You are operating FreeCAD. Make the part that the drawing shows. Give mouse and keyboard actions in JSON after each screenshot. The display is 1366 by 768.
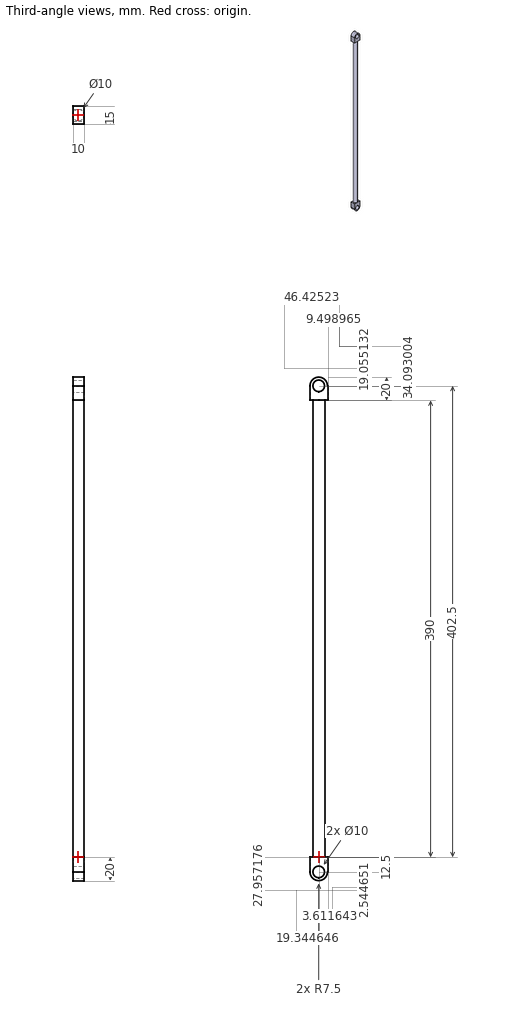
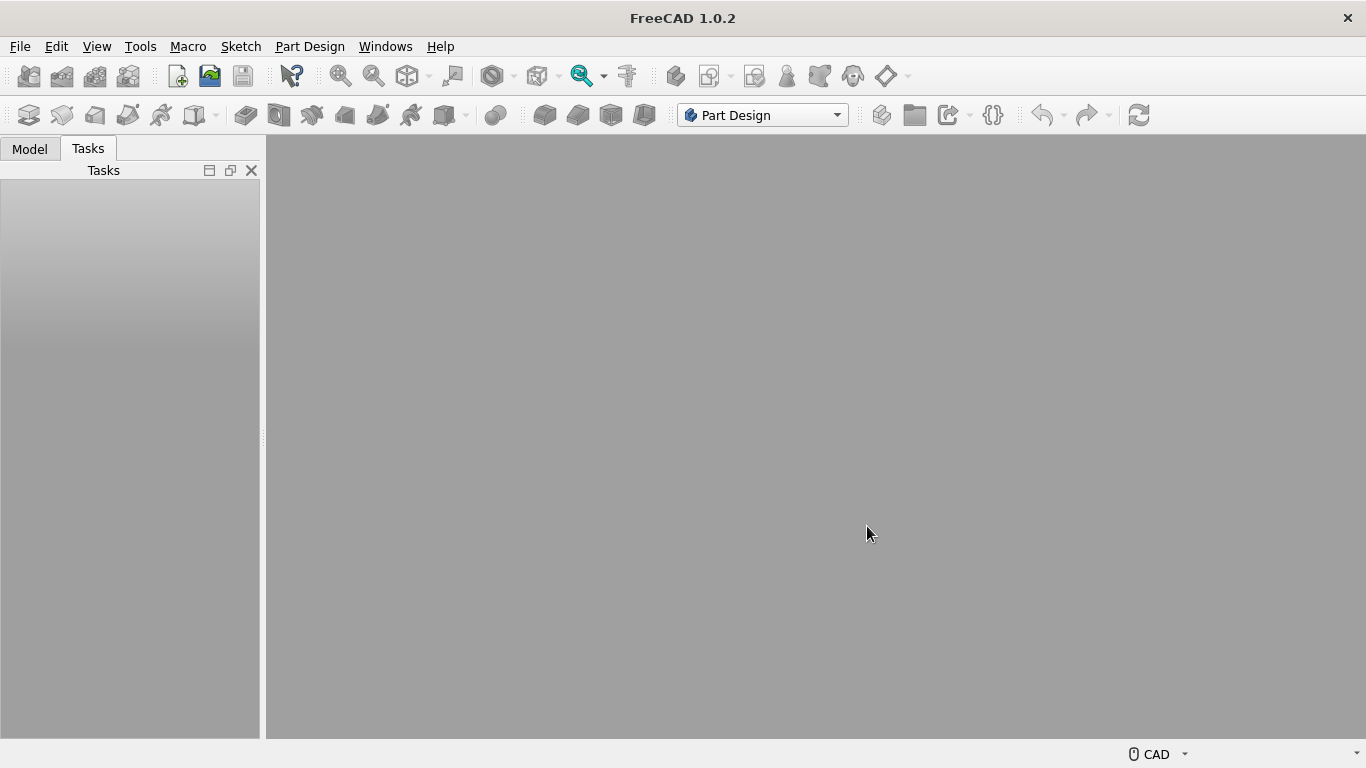
{"action": "left_click", "coordinate": [177, 76]}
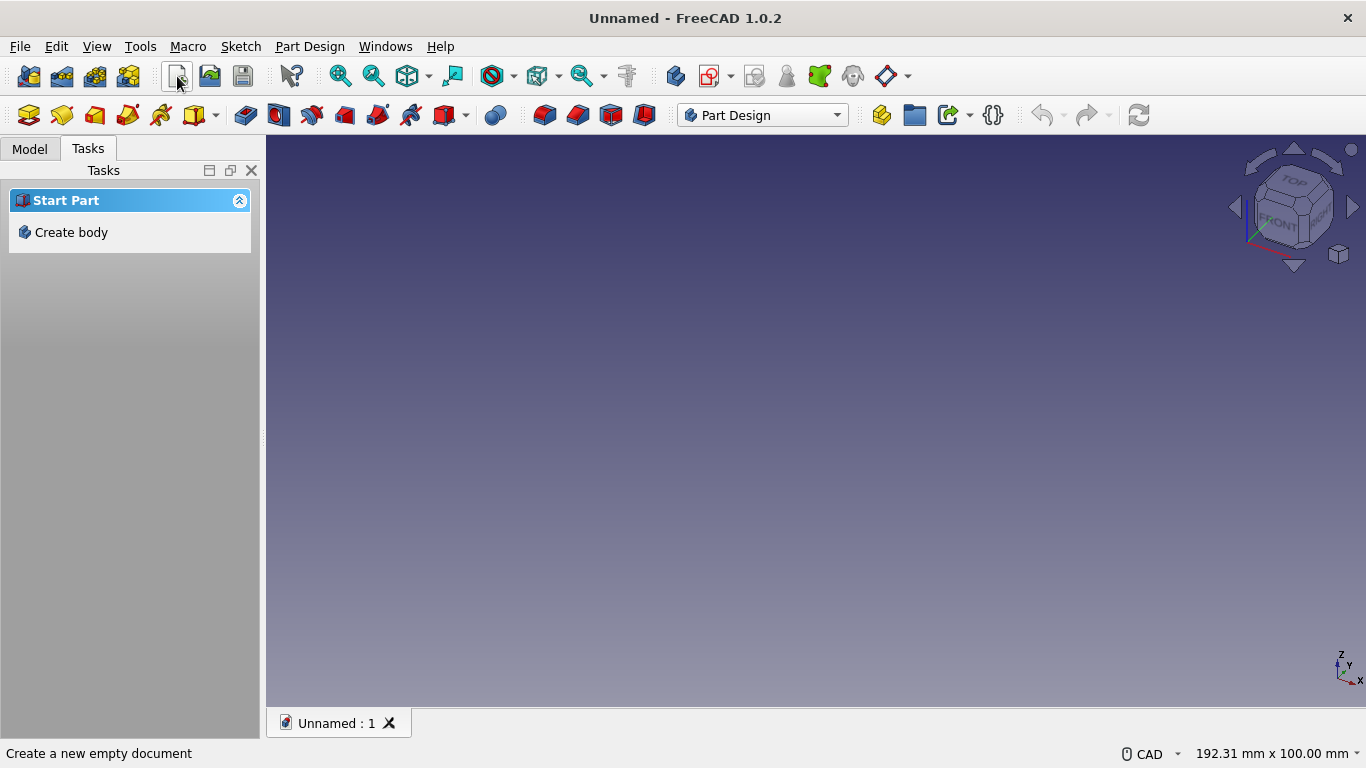
{"action": "left_click", "coordinate": [708, 76]}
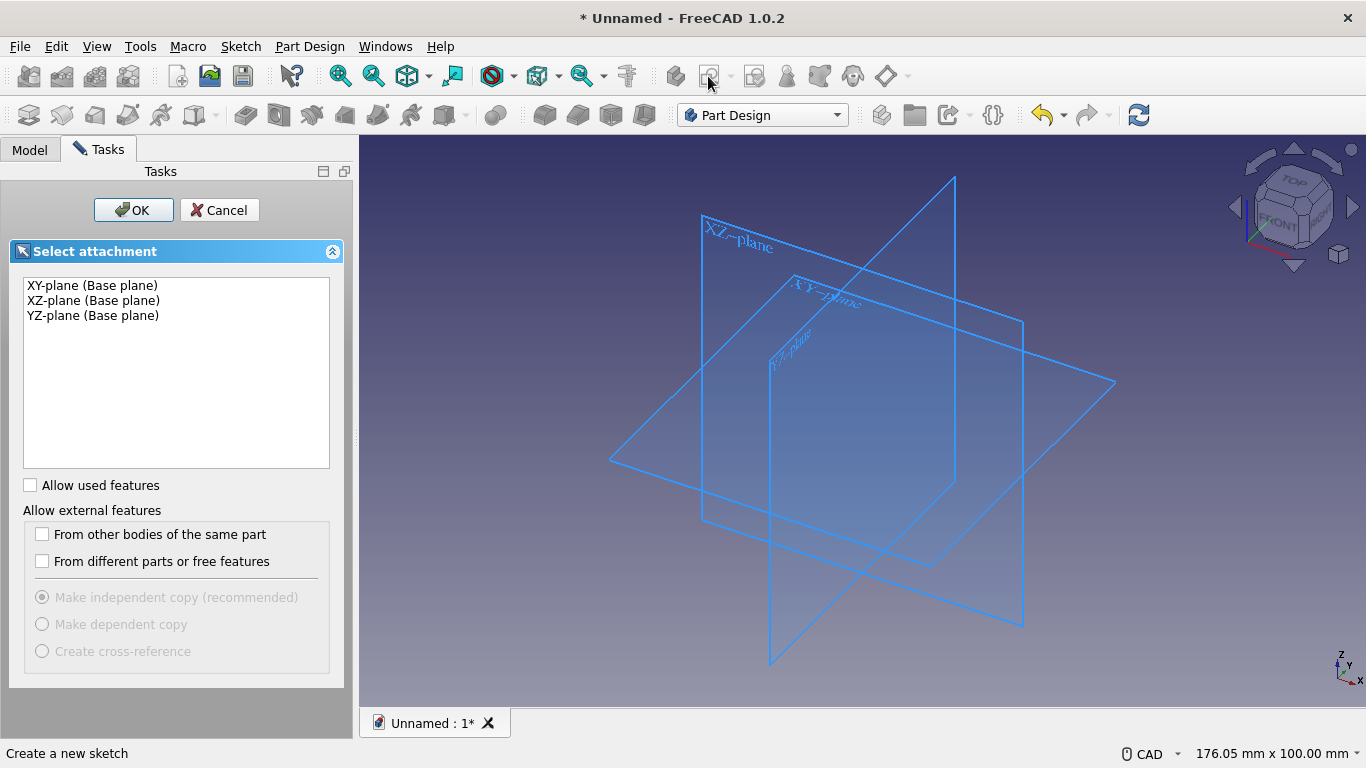
{"action": "left_click", "coordinate": [84, 286]}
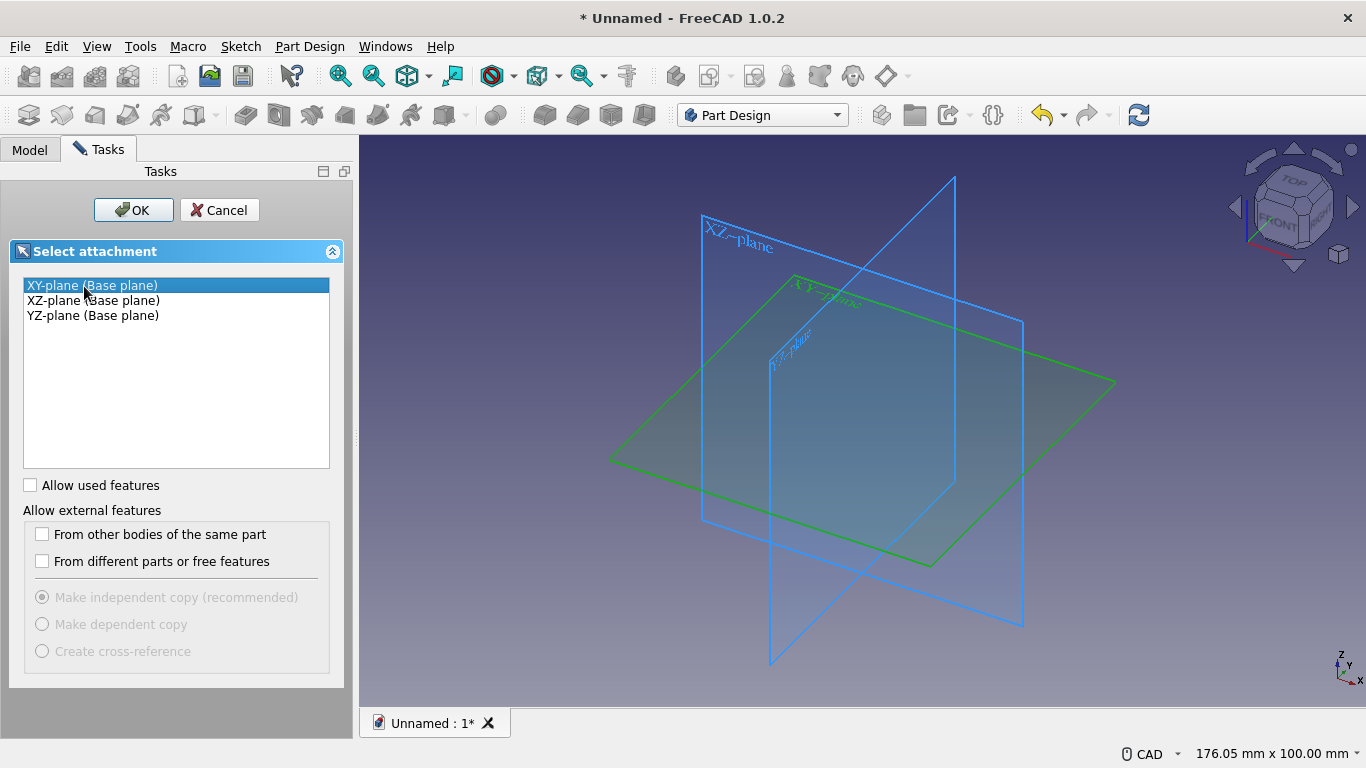
{"action": "left_click", "coordinate": [134, 210]}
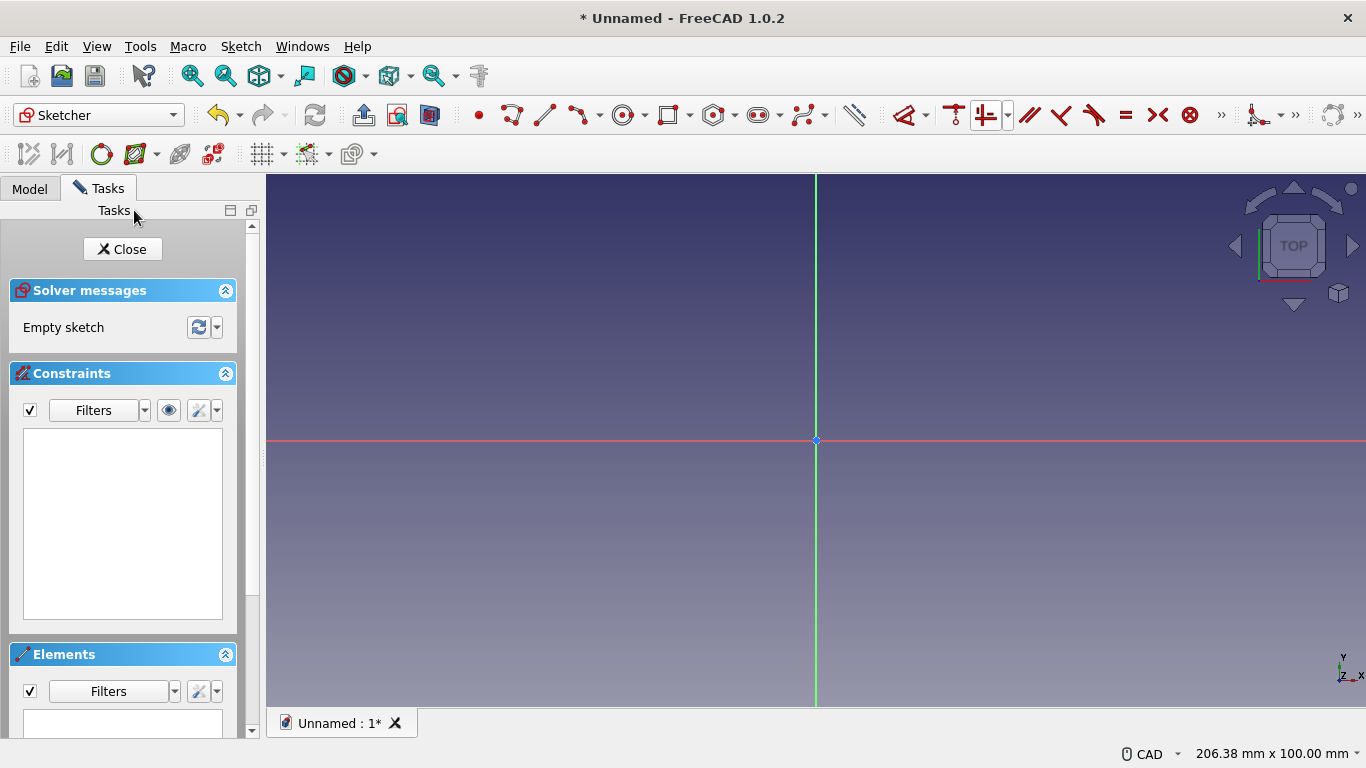
{"action": "scroll", "coordinate": [830, 440], "scroll_direction": "up", "scroll_amount": 9}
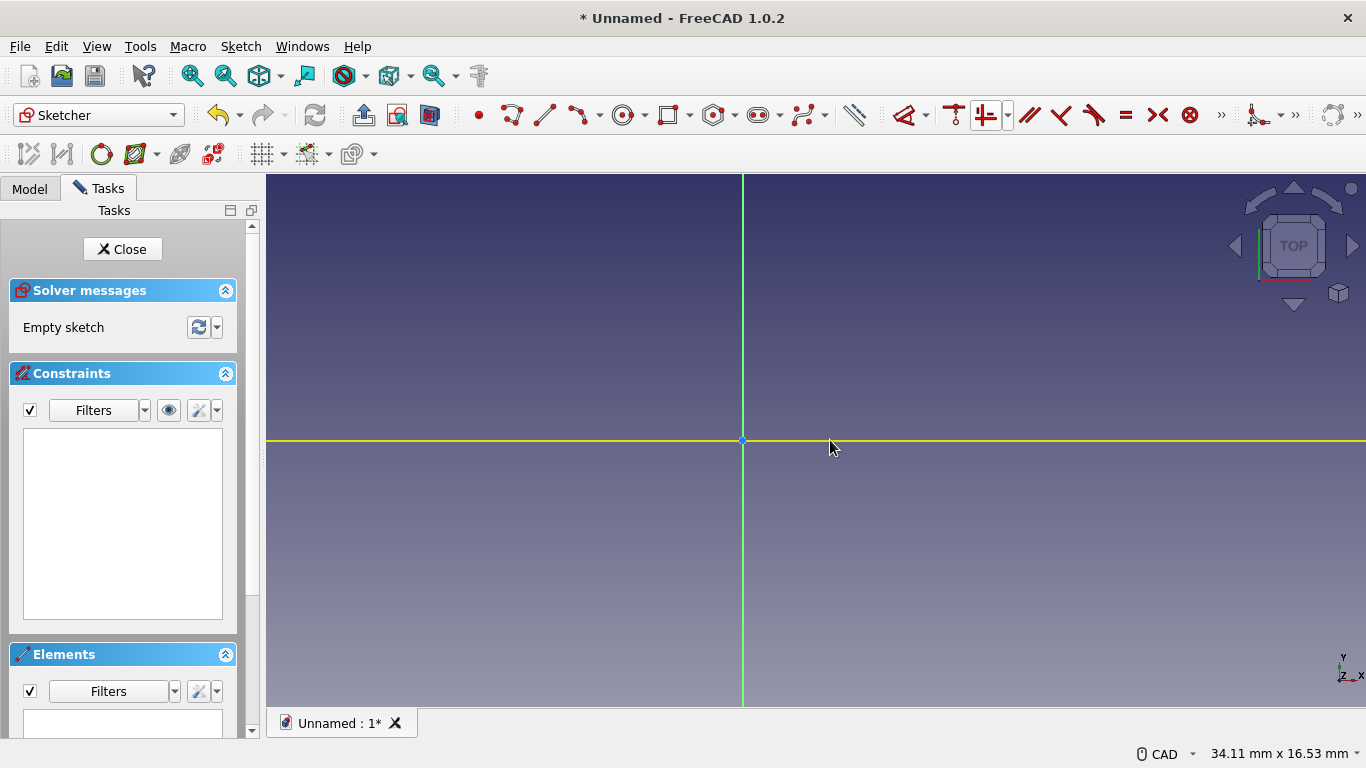
{"action": "left_click", "coordinate": [622, 116]}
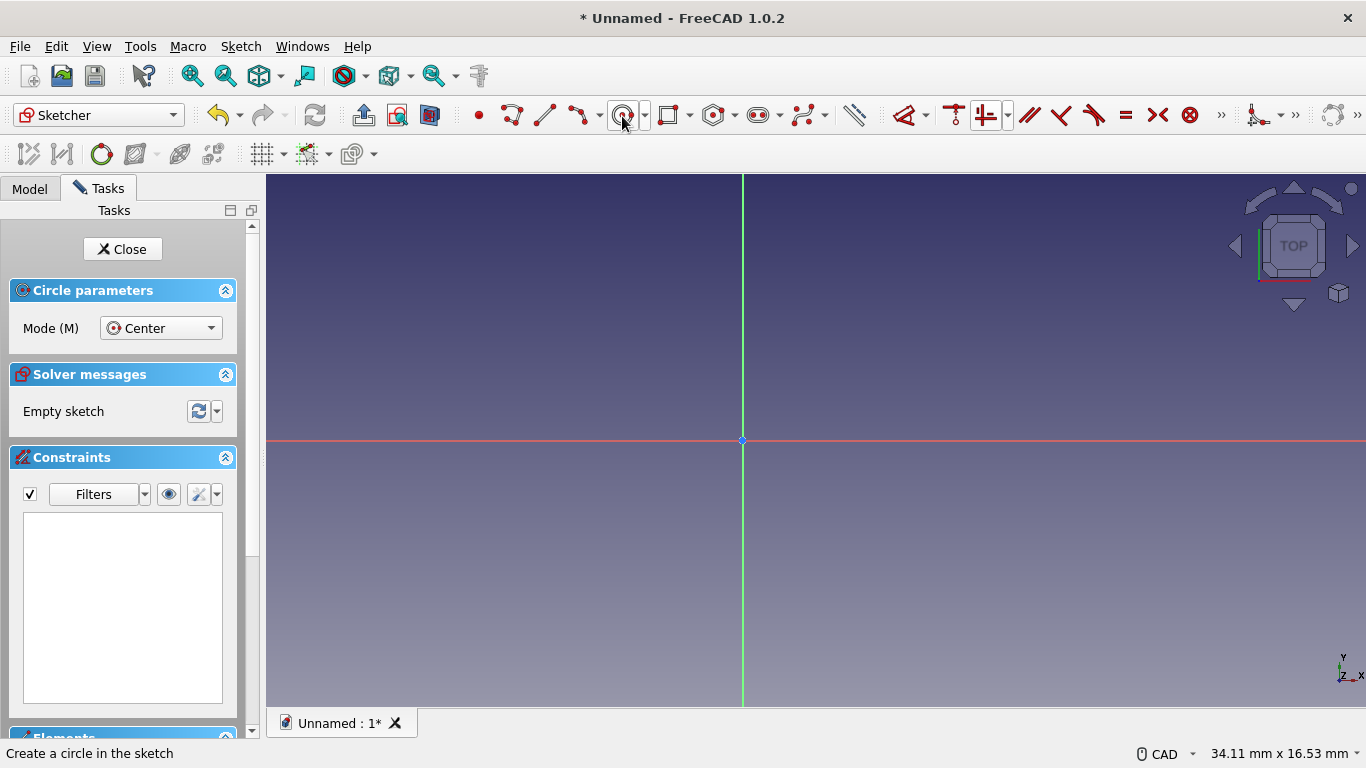
{"action": "left_click", "coordinate": [743, 440]}
{"action": "mouse_move", "coordinate": [857, 326]}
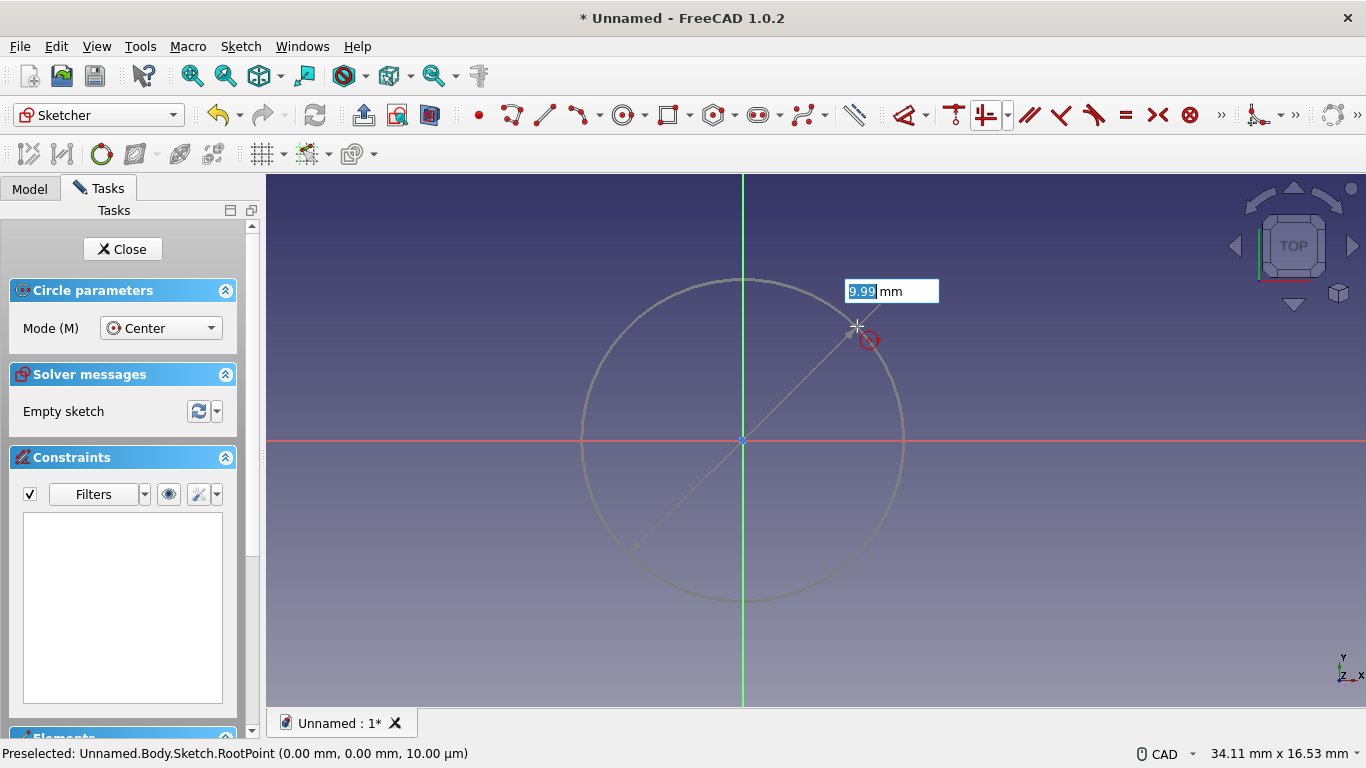
{"action": "type", "text": "10"}
{"action": "key", "text": "Return"}
{"action": "key", "text": "Escape"}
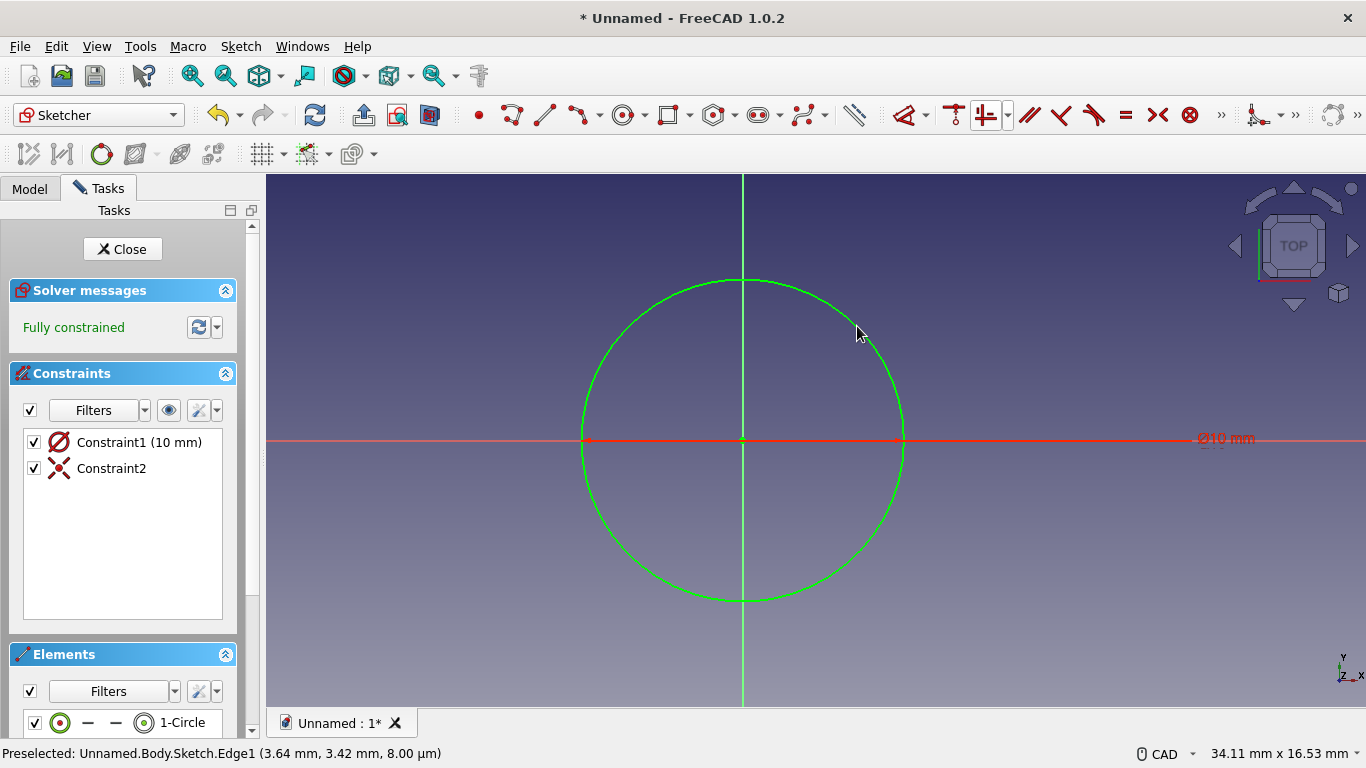
{"action": "left_click", "coordinate": [123, 249]}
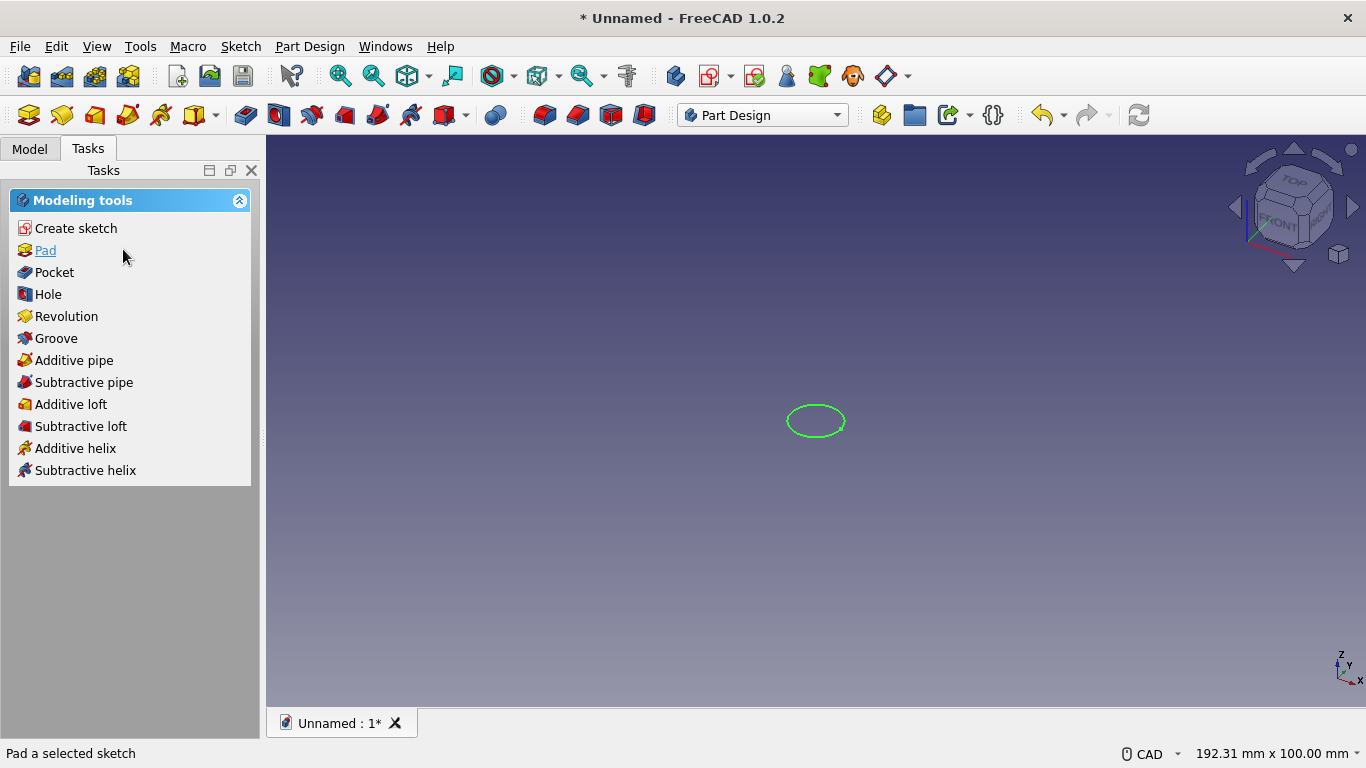
{"action": "left_click", "coordinate": [29, 116]}